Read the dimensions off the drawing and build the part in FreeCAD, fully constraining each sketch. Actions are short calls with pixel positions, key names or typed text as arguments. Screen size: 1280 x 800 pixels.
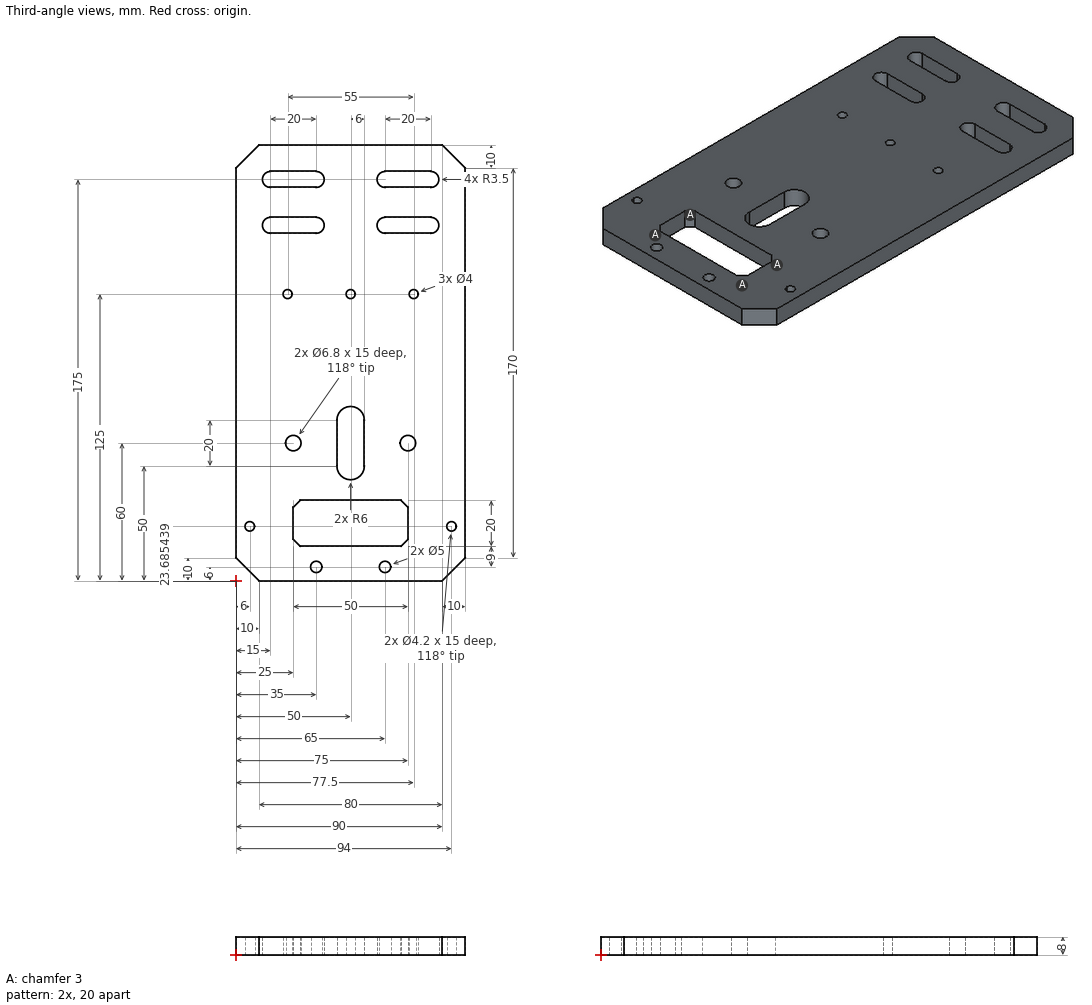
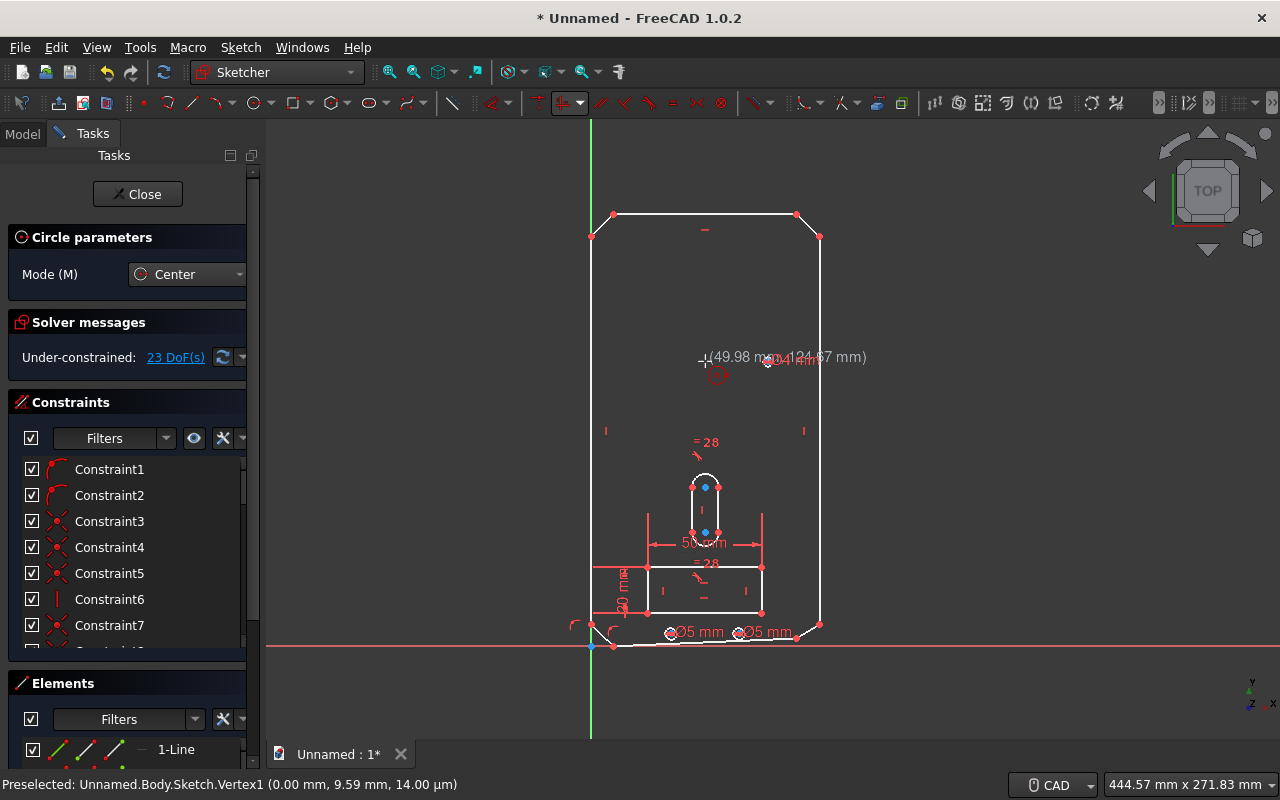
click(705, 361)
move(708, 358)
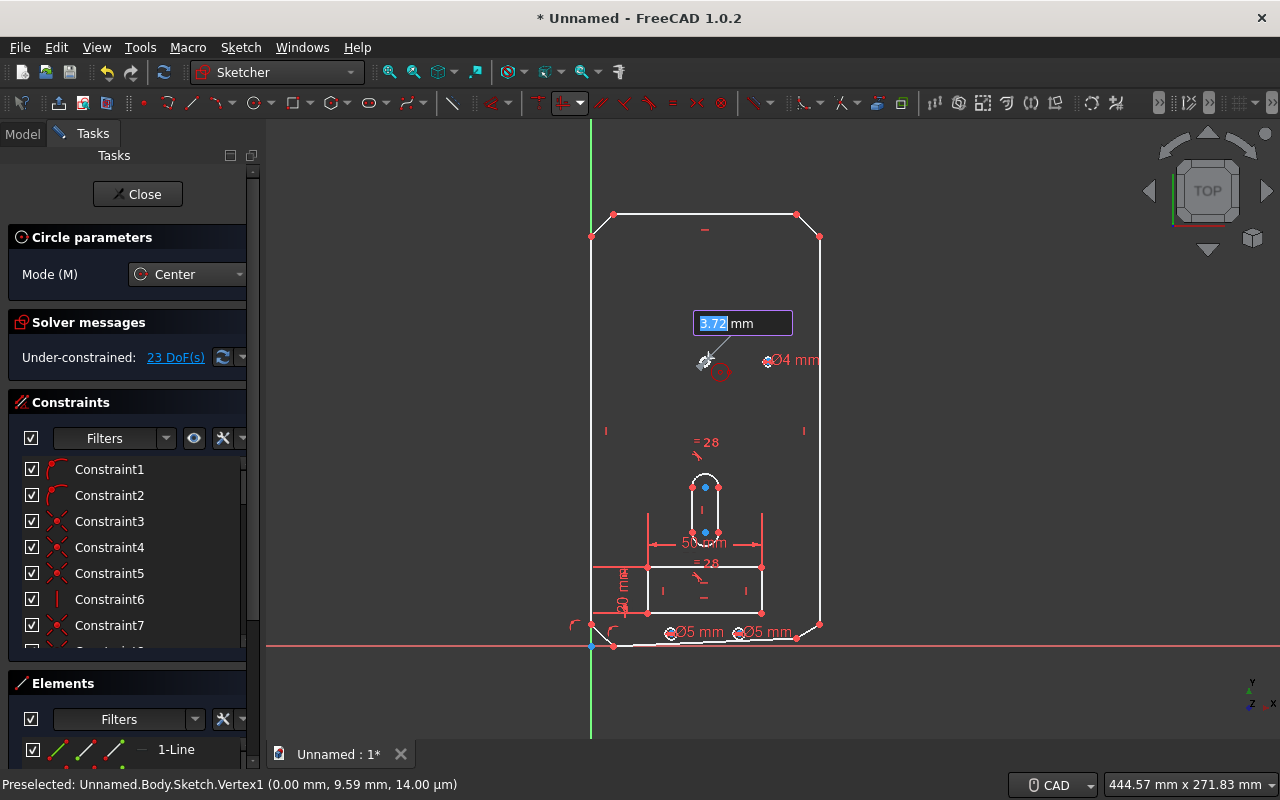
text(4)
key(Return)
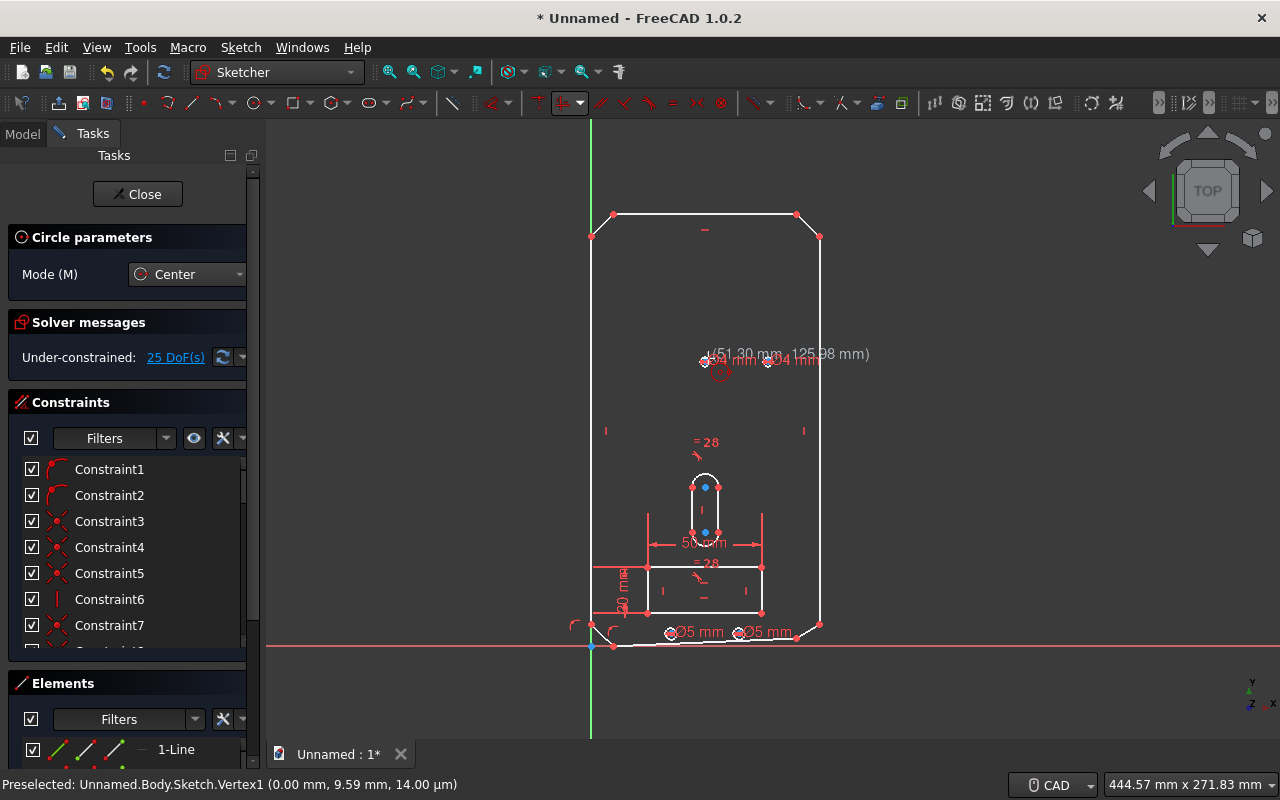
scroll(642, 361, up, 9)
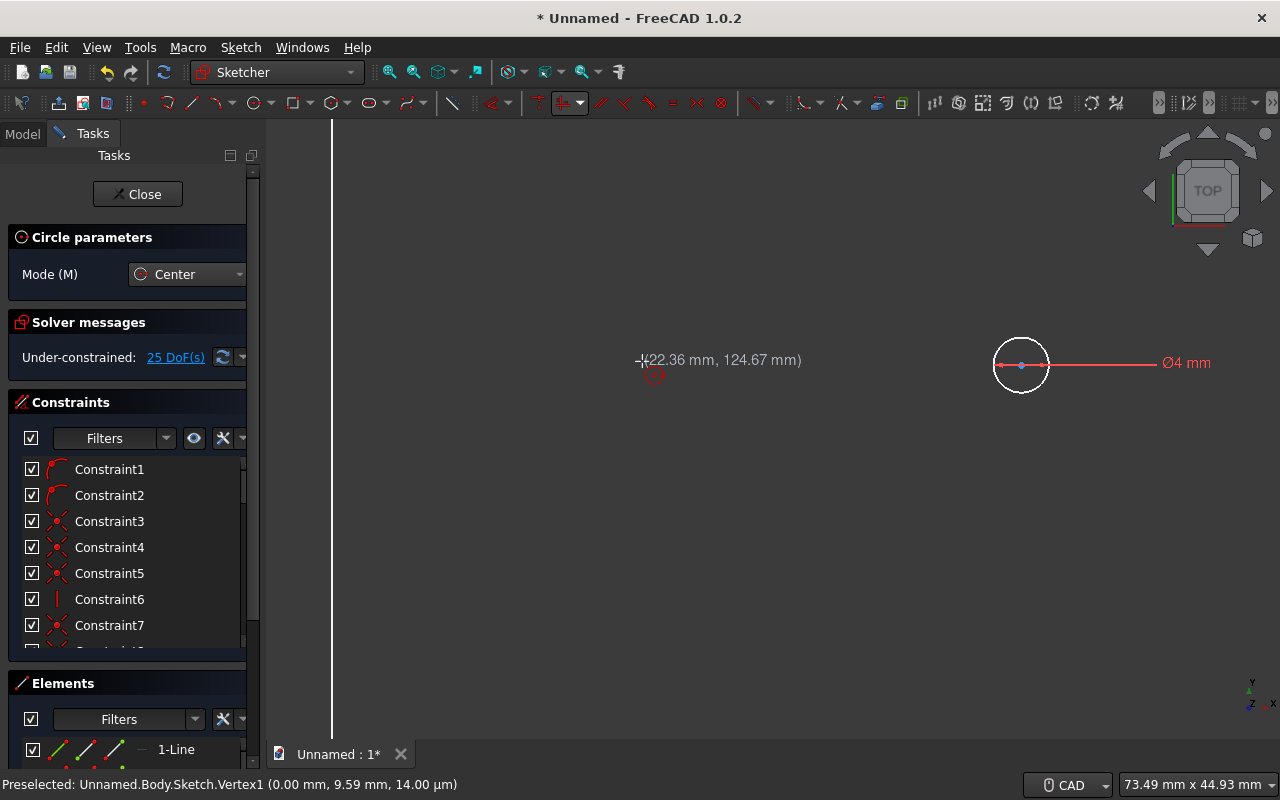
scroll(642, 361, down, 9)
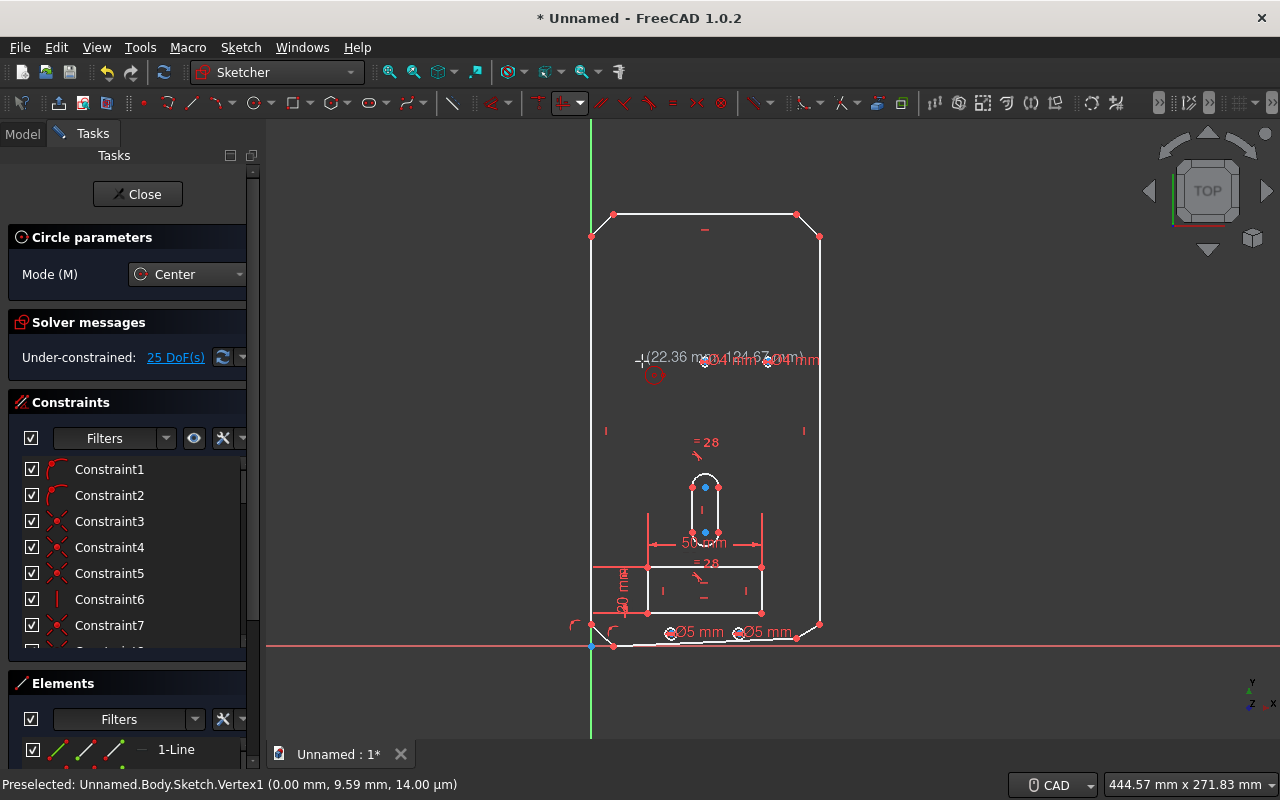
click(642, 361)
move(646, 358)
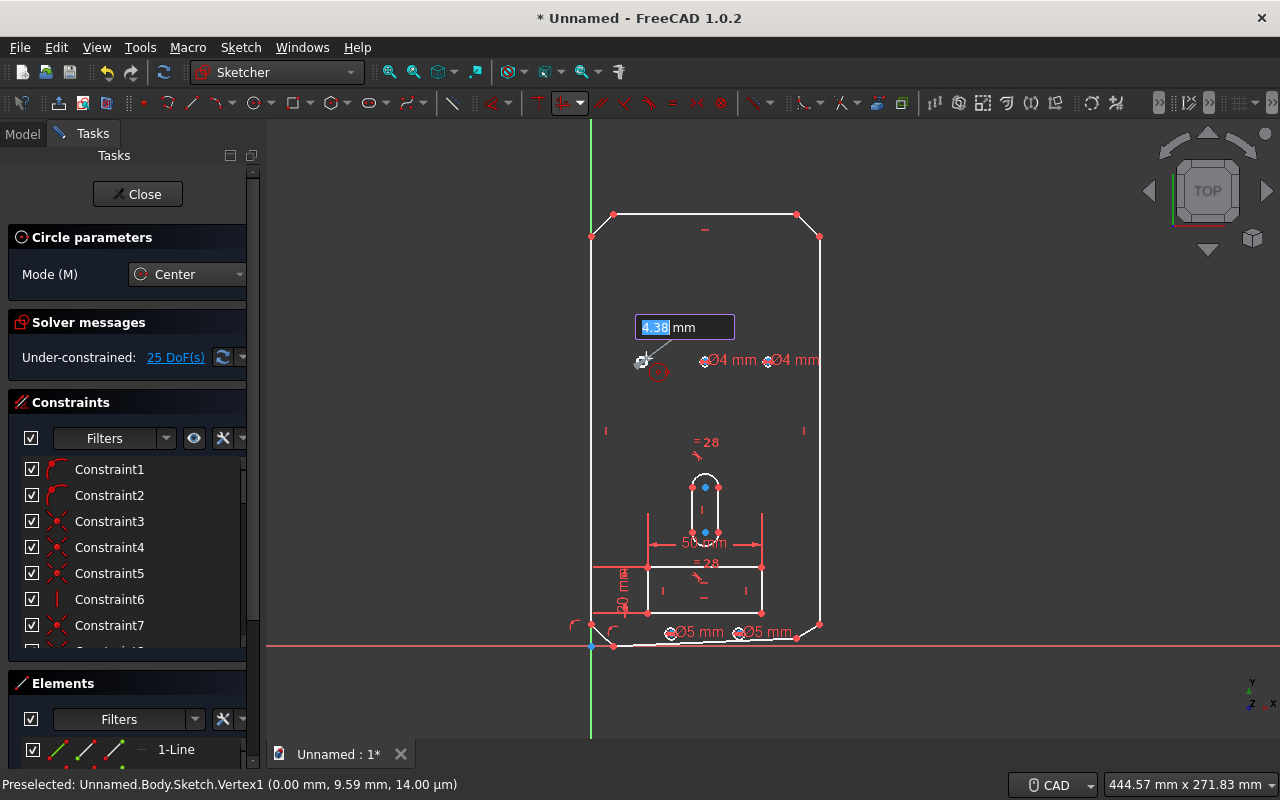
text(4)
key(Return)
key(Escape)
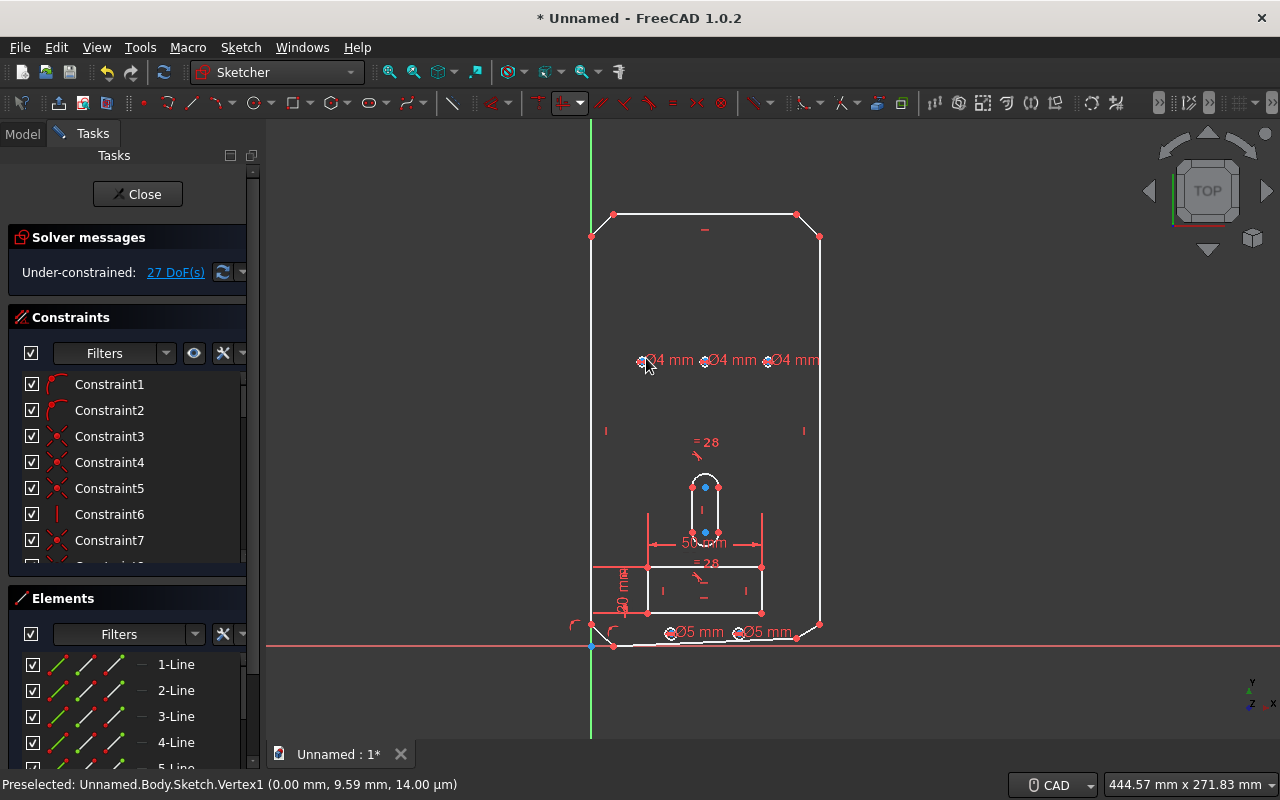
click(687, 643)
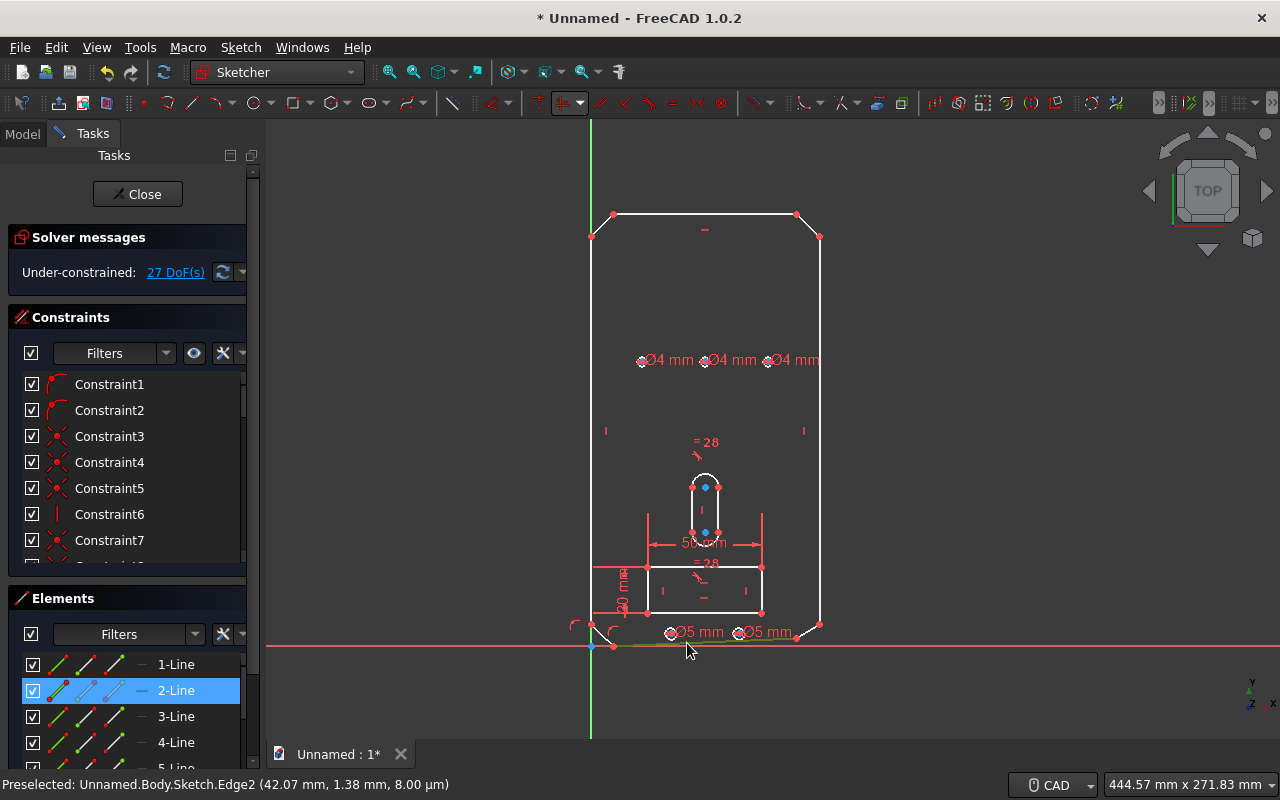
key(h)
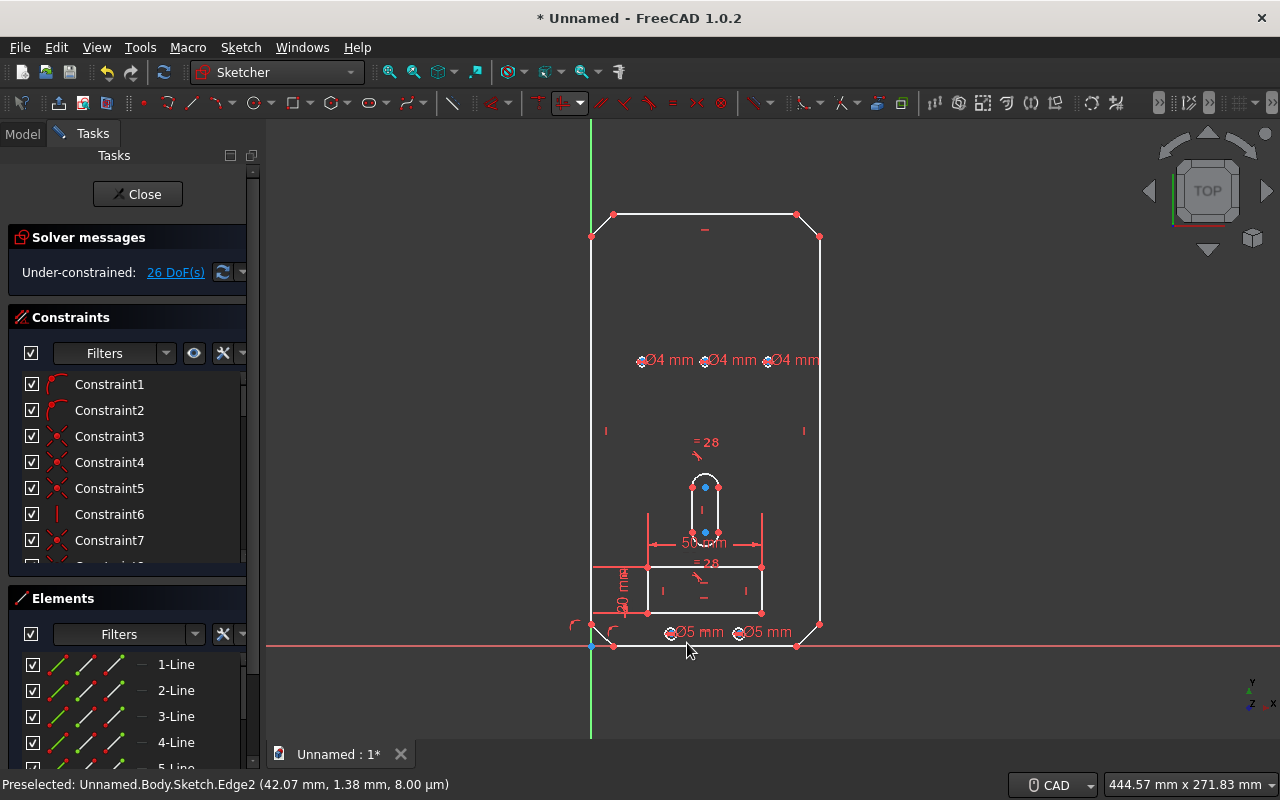
click(739, 634)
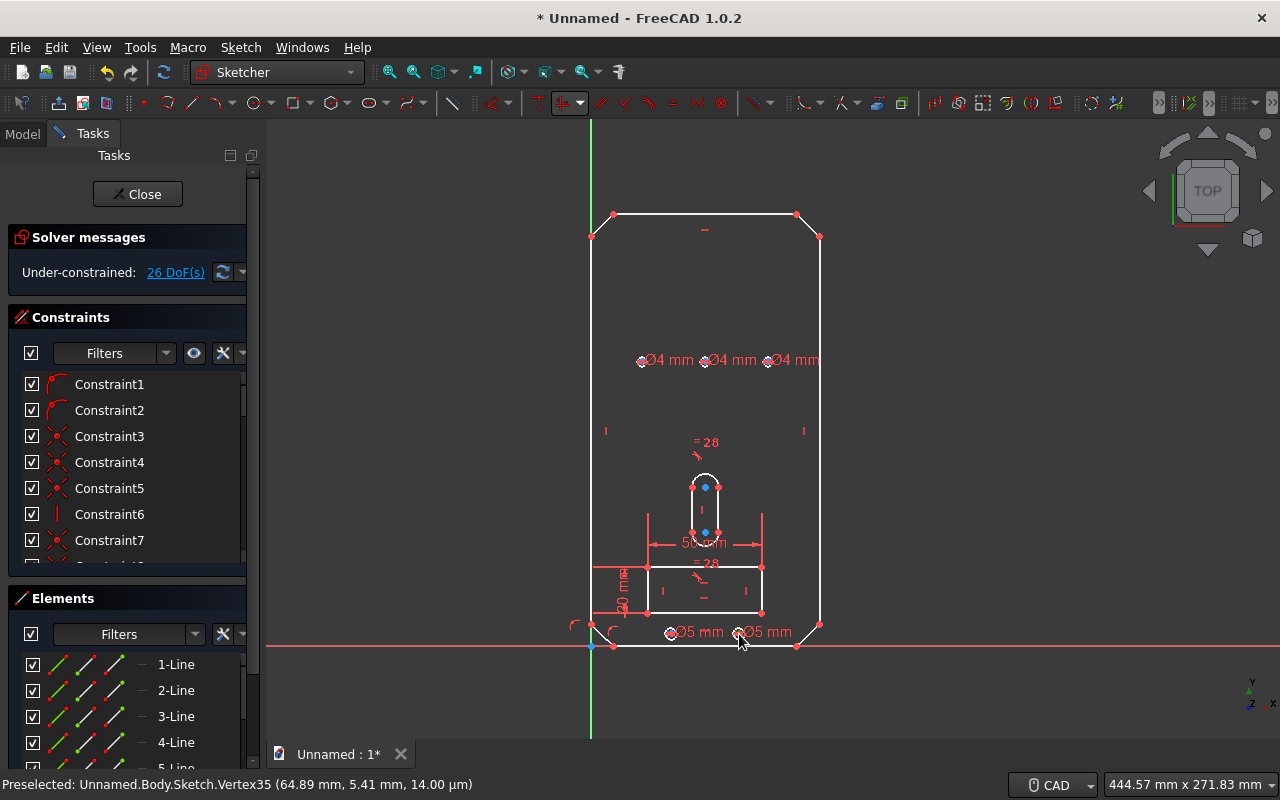
click(671, 634)